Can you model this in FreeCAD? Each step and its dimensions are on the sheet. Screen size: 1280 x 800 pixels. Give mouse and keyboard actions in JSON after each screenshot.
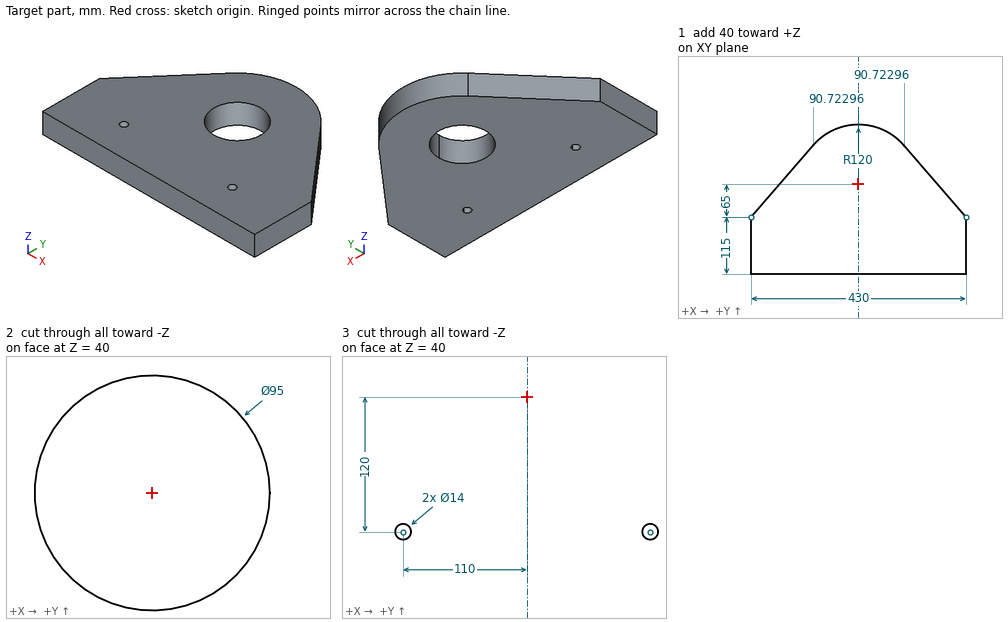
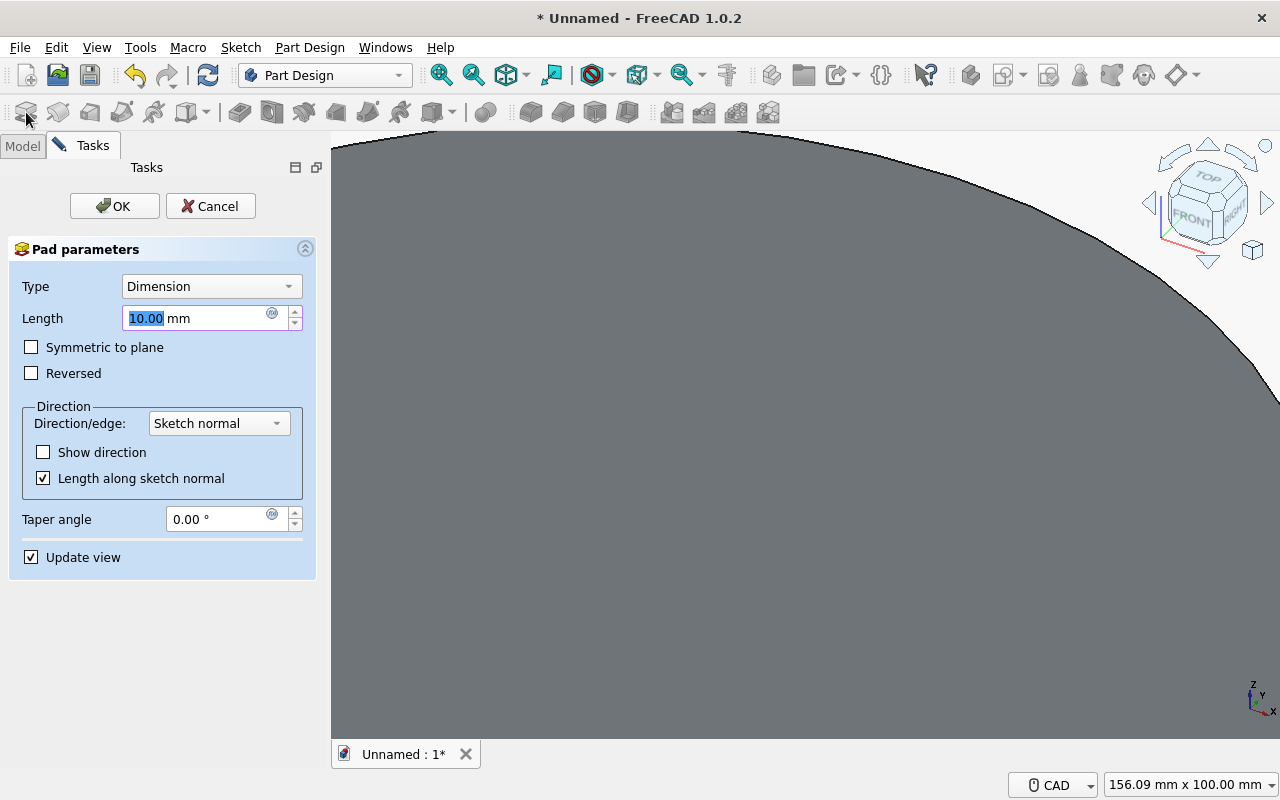
{"action": "type", "text": "40"}
{"action": "key", "text": "Tab"}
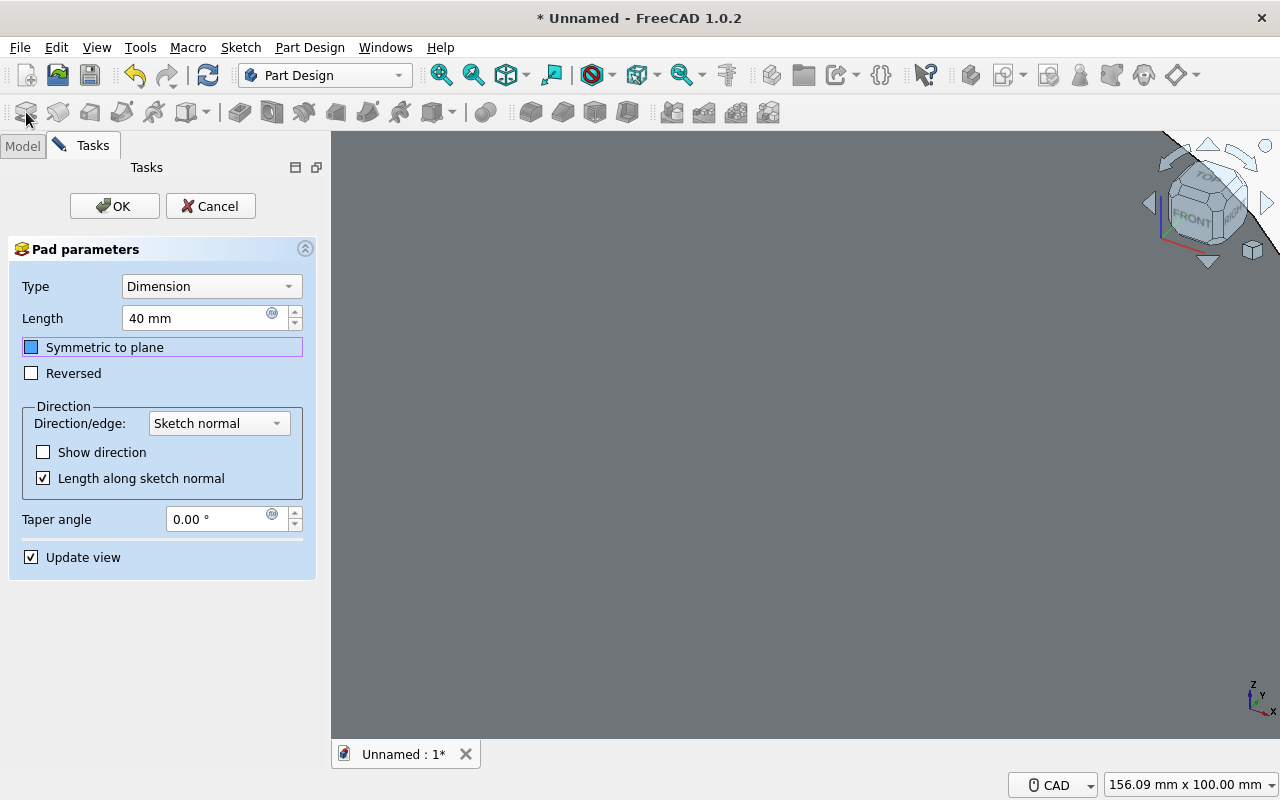
{"action": "left_click", "coordinate": [115, 206]}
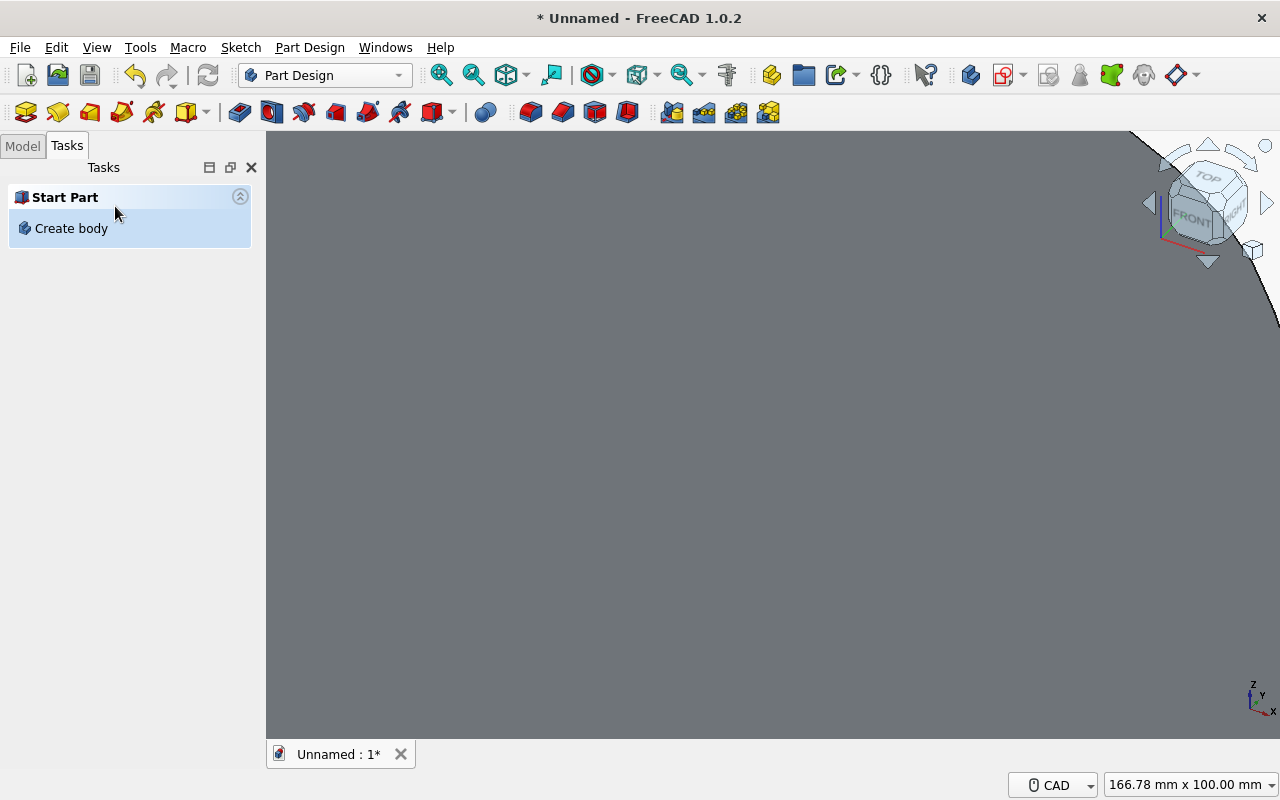
{"action": "left_click", "coordinate": [442, 76]}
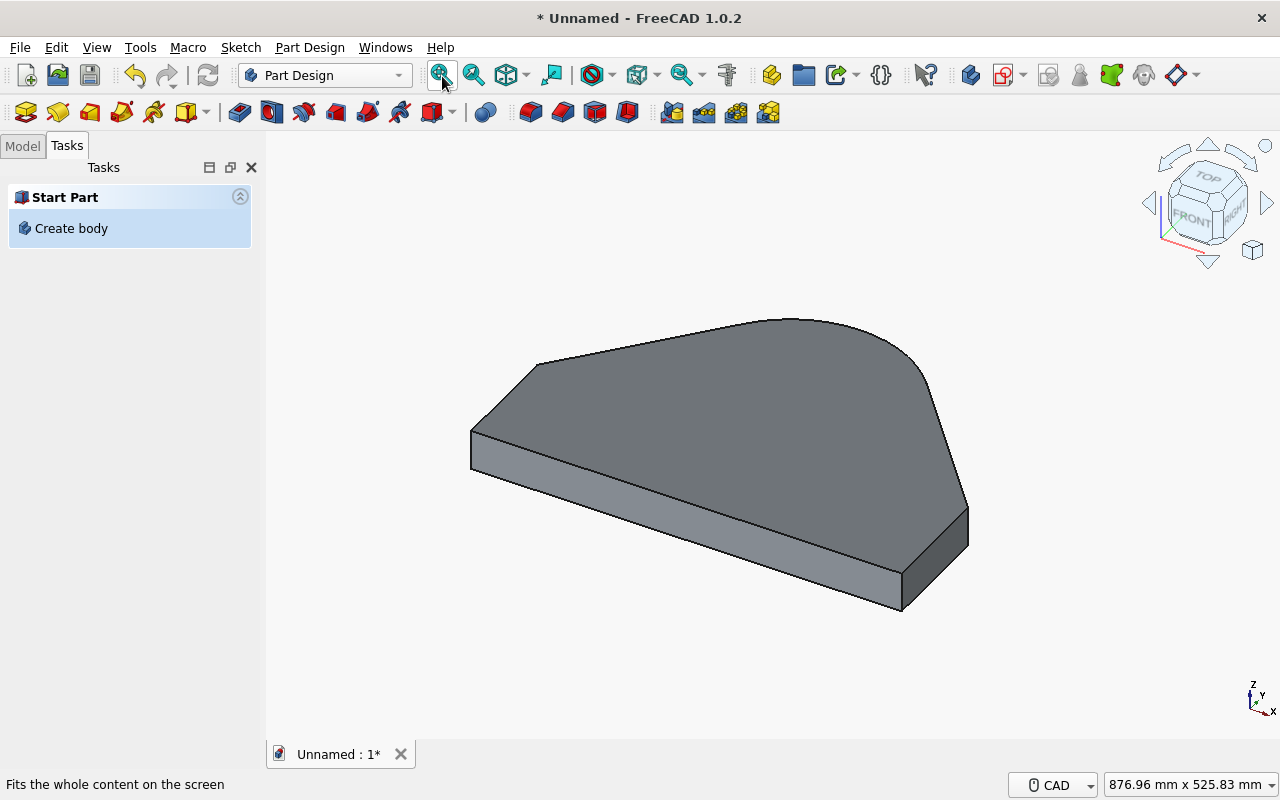
{"action": "left_click", "coordinate": [773, 415]}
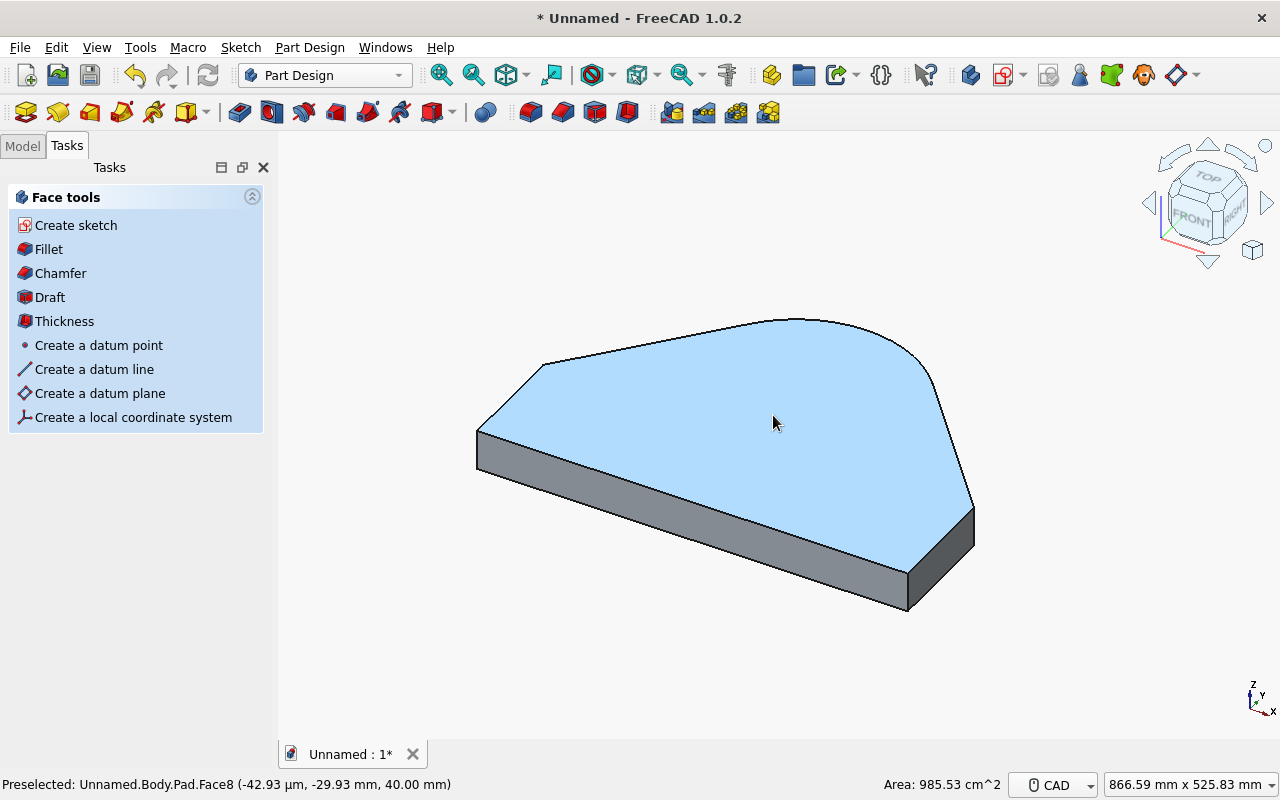
{"action": "left_click", "coordinate": [1004, 76]}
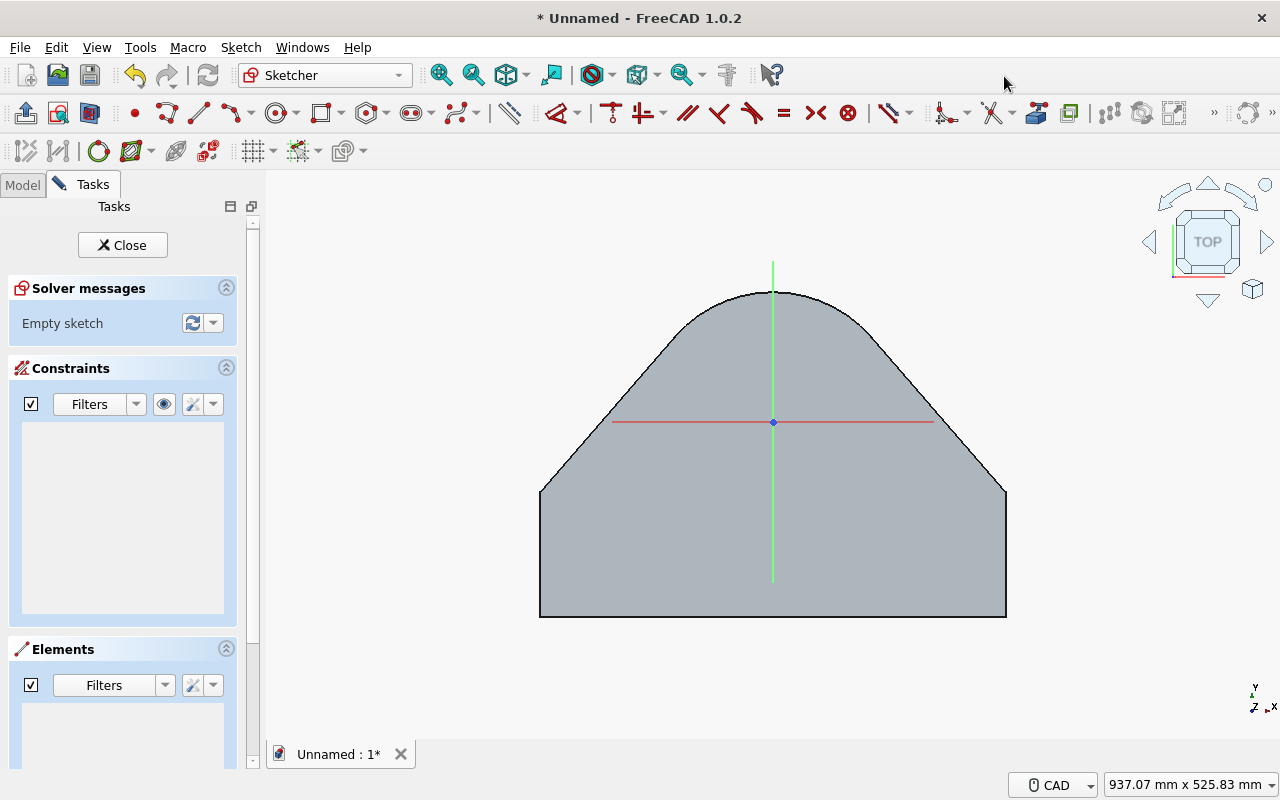
{"action": "scroll", "coordinate": [803, 408], "scroll_direction": "up", "scroll_amount": 6}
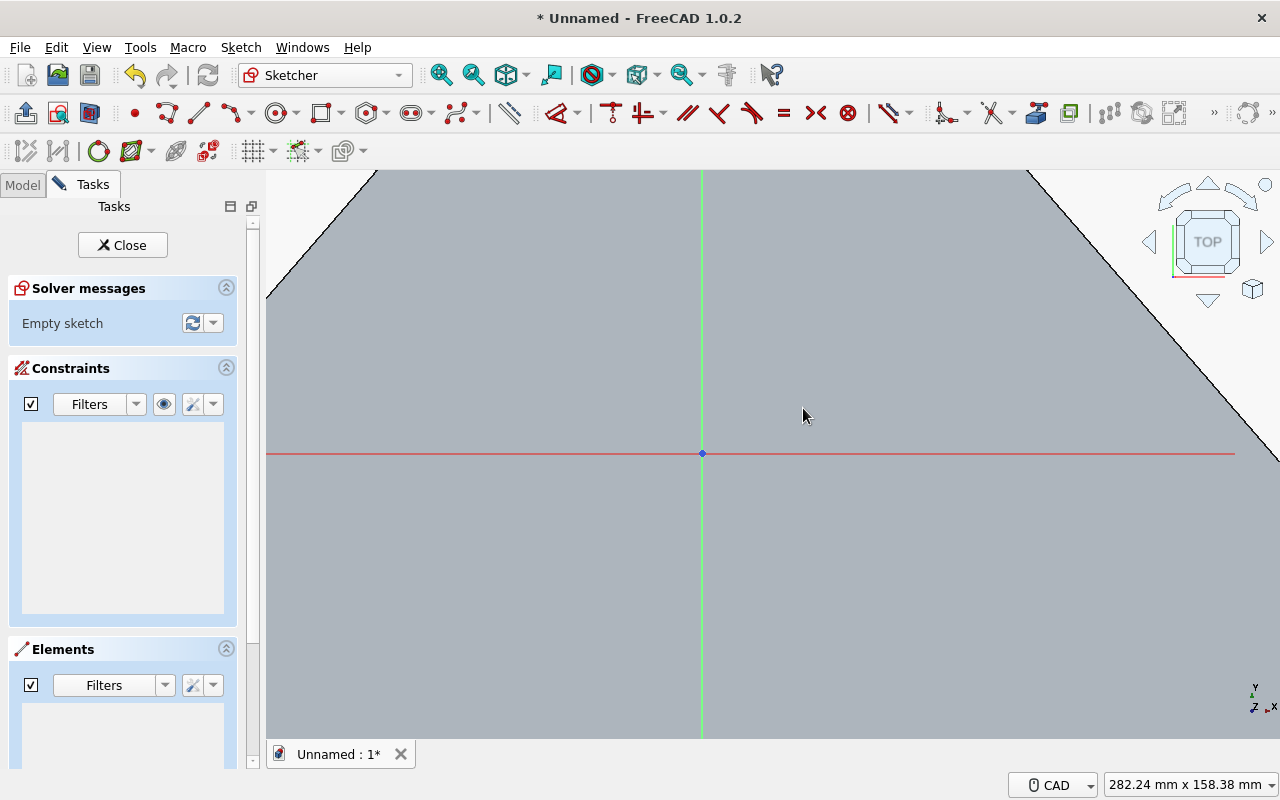
{"action": "left_click", "coordinate": [276, 114]}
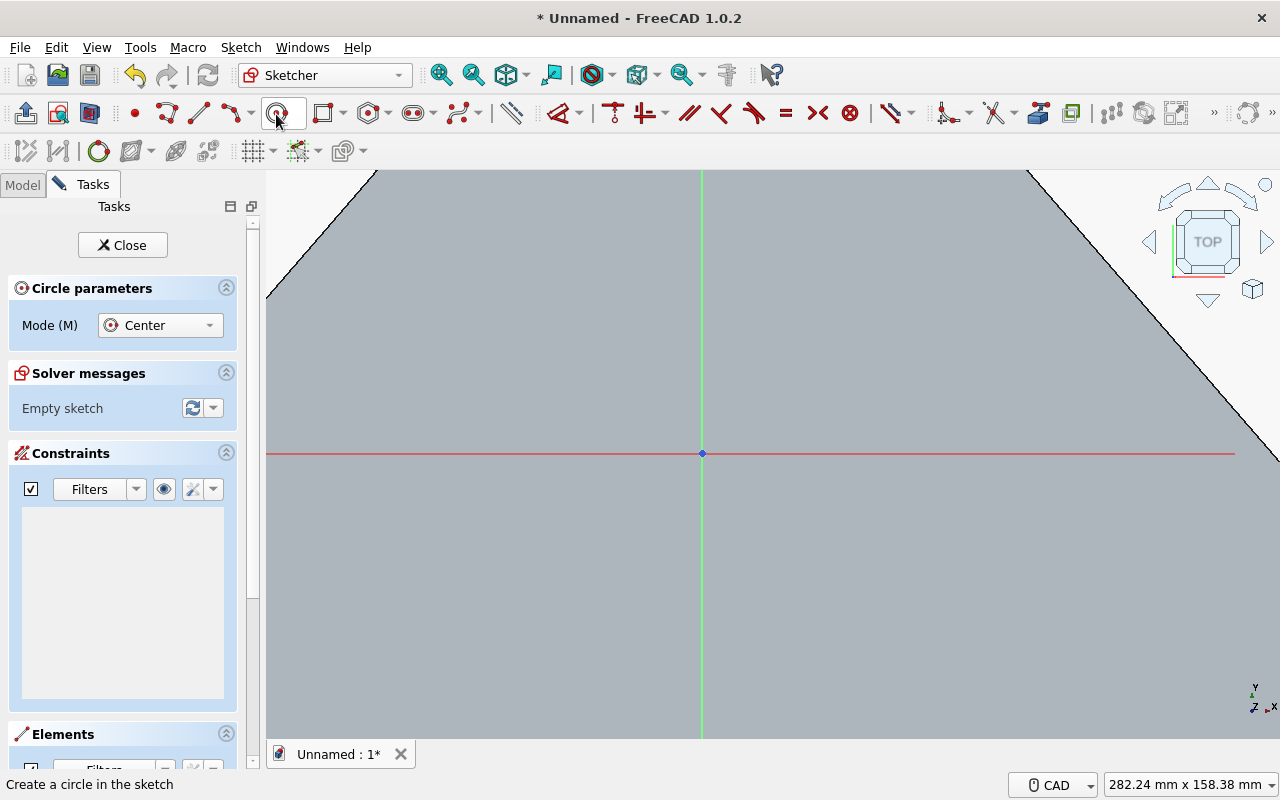
{"action": "left_click", "coordinate": [702, 454]}
{"action": "mouse_move", "coordinate": [823, 333]}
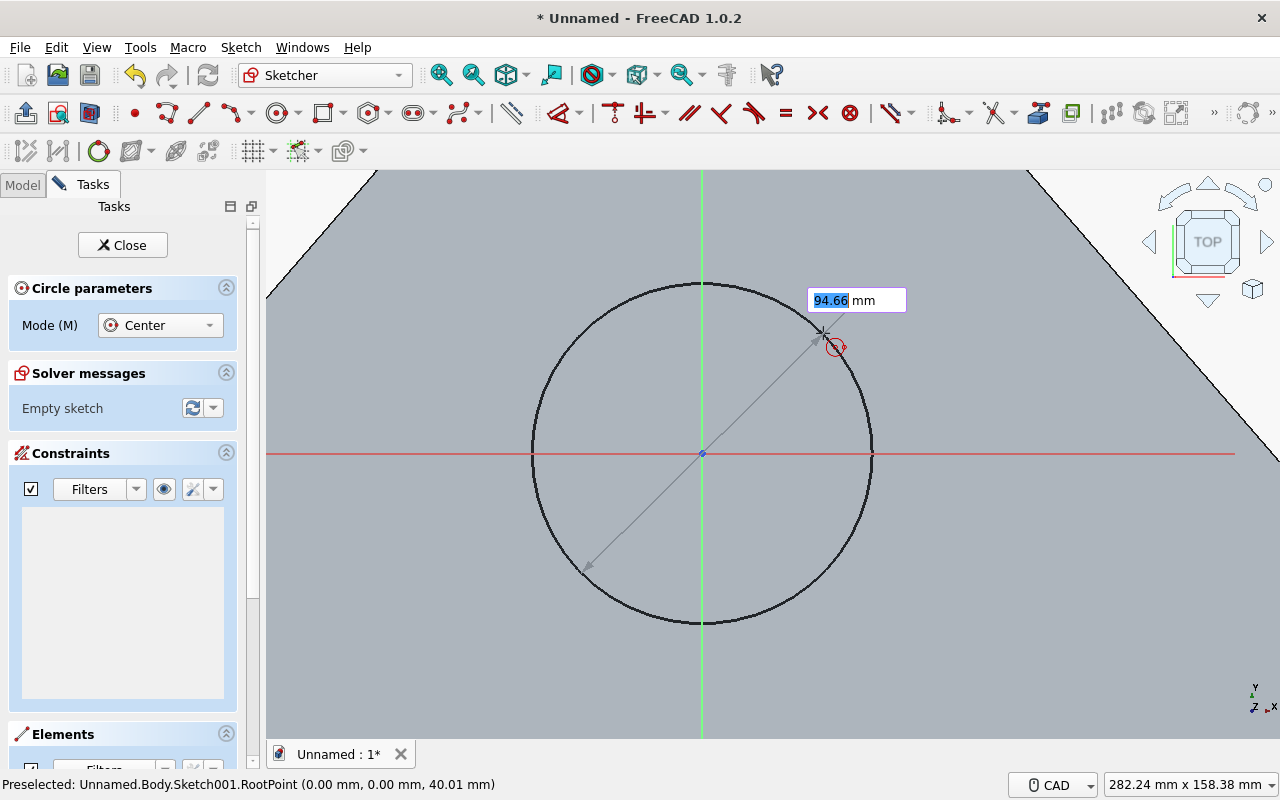
{"action": "type", "text": "95"}
{"action": "key", "text": "Return"}
{"action": "key", "text": "Escape"}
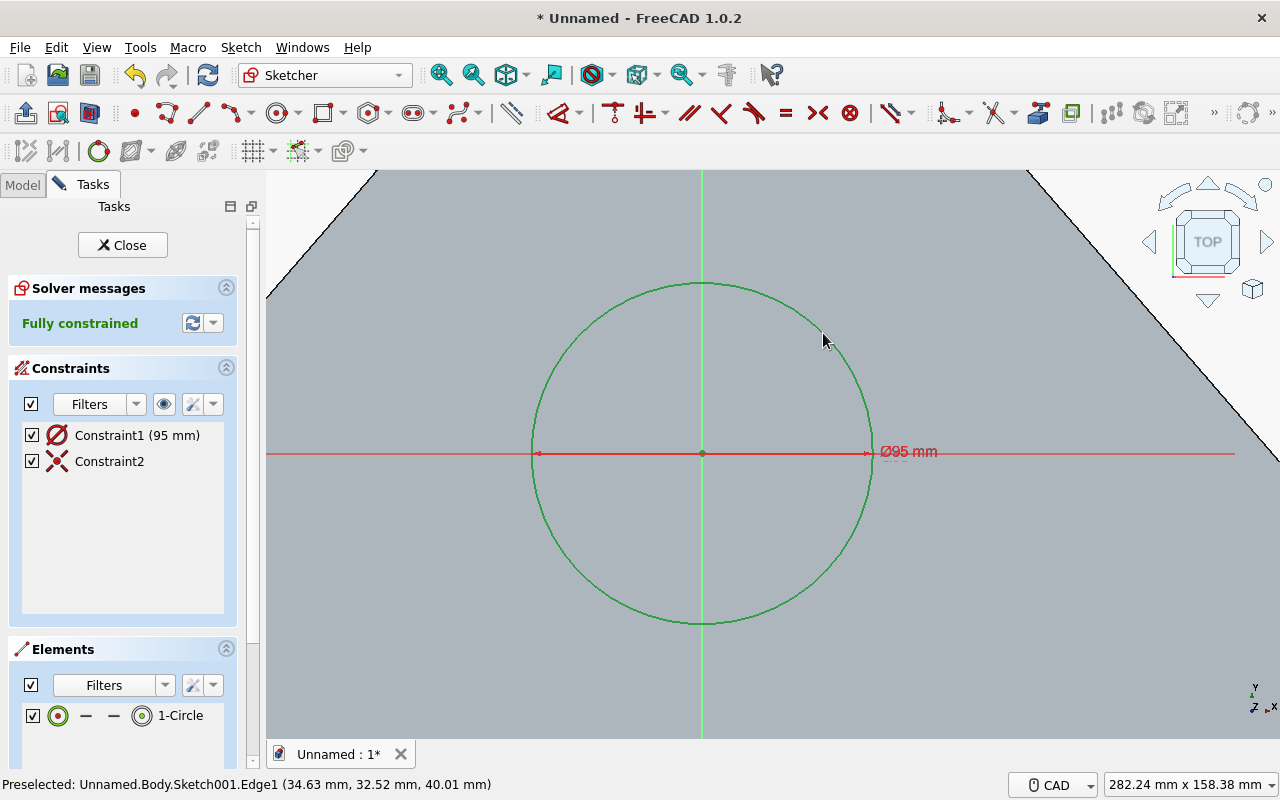
{"action": "left_click", "coordinate": [123, 245]}